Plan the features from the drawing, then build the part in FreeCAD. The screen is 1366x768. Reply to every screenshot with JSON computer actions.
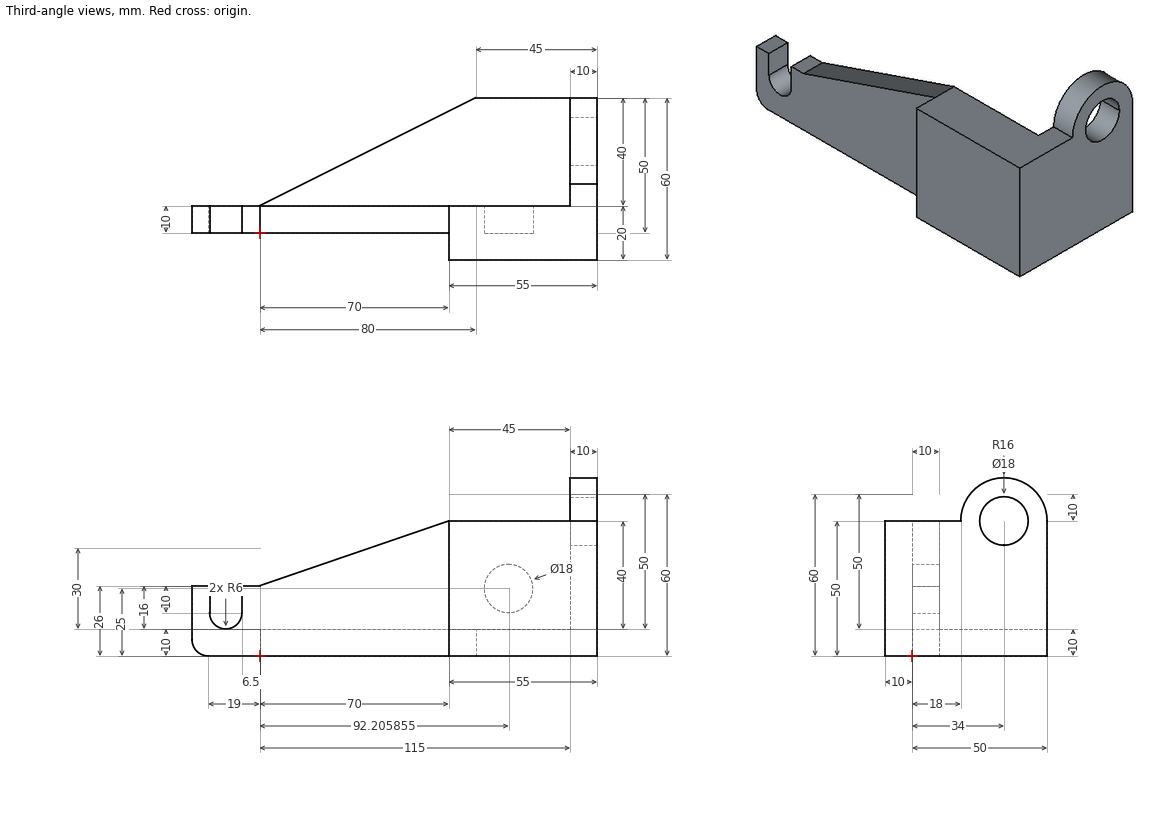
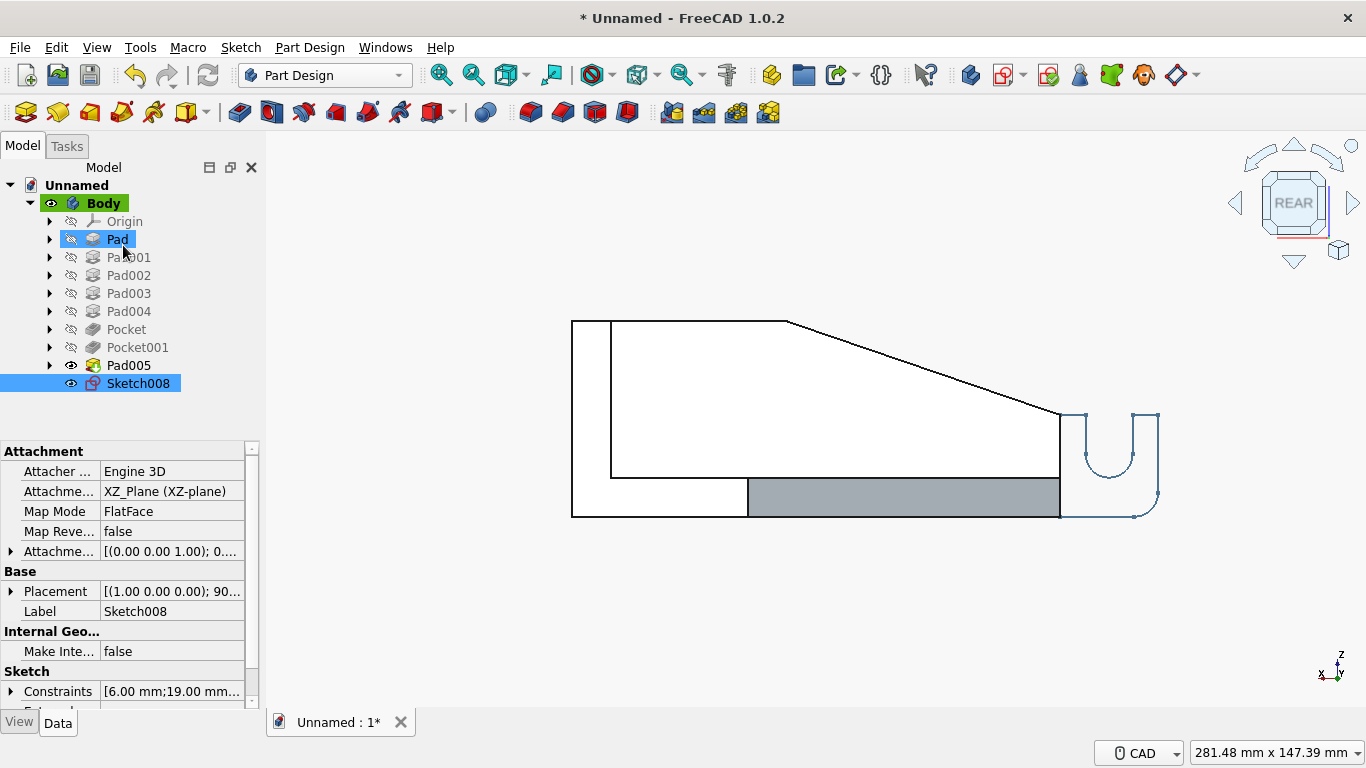
{"action": "left_click", "coordinate": [26, 112]}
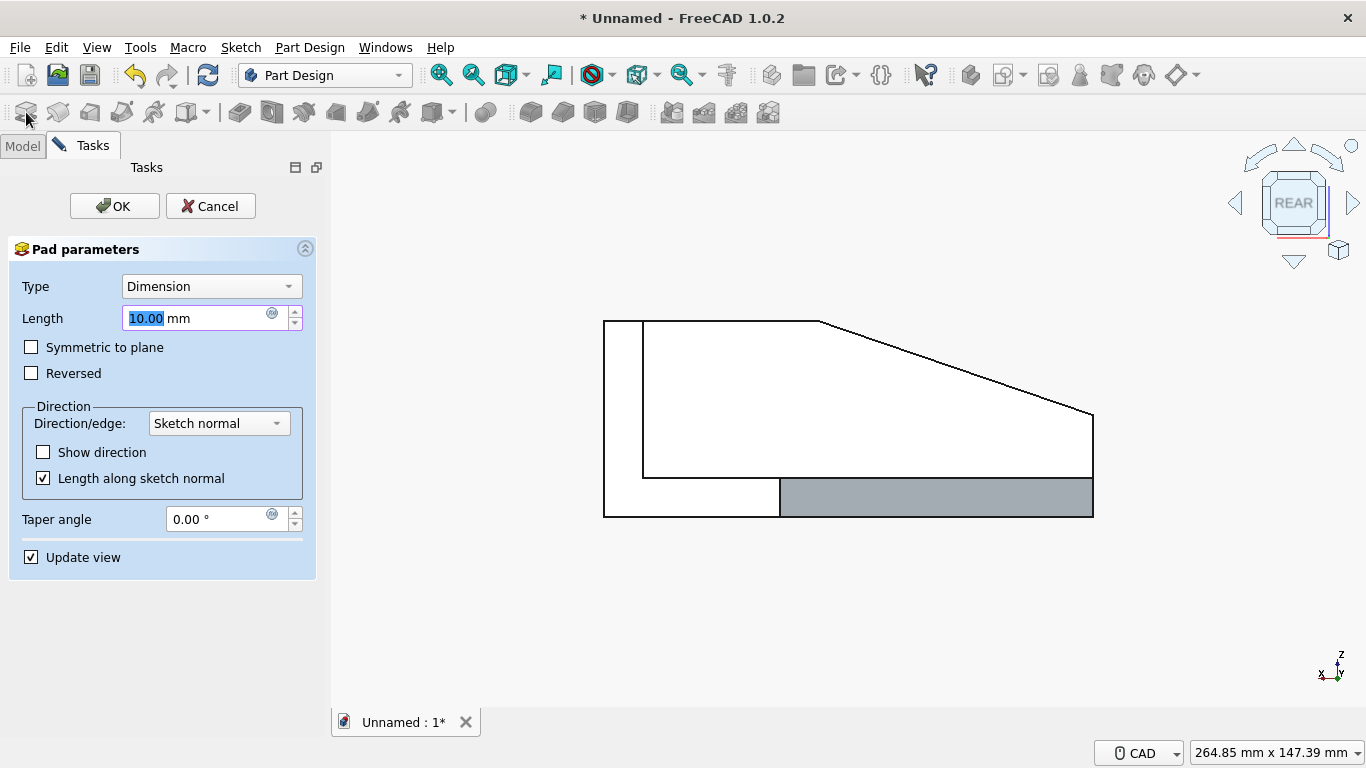
{"action": "type", "text": "10"}
{"action": "key", "text": "Tab"}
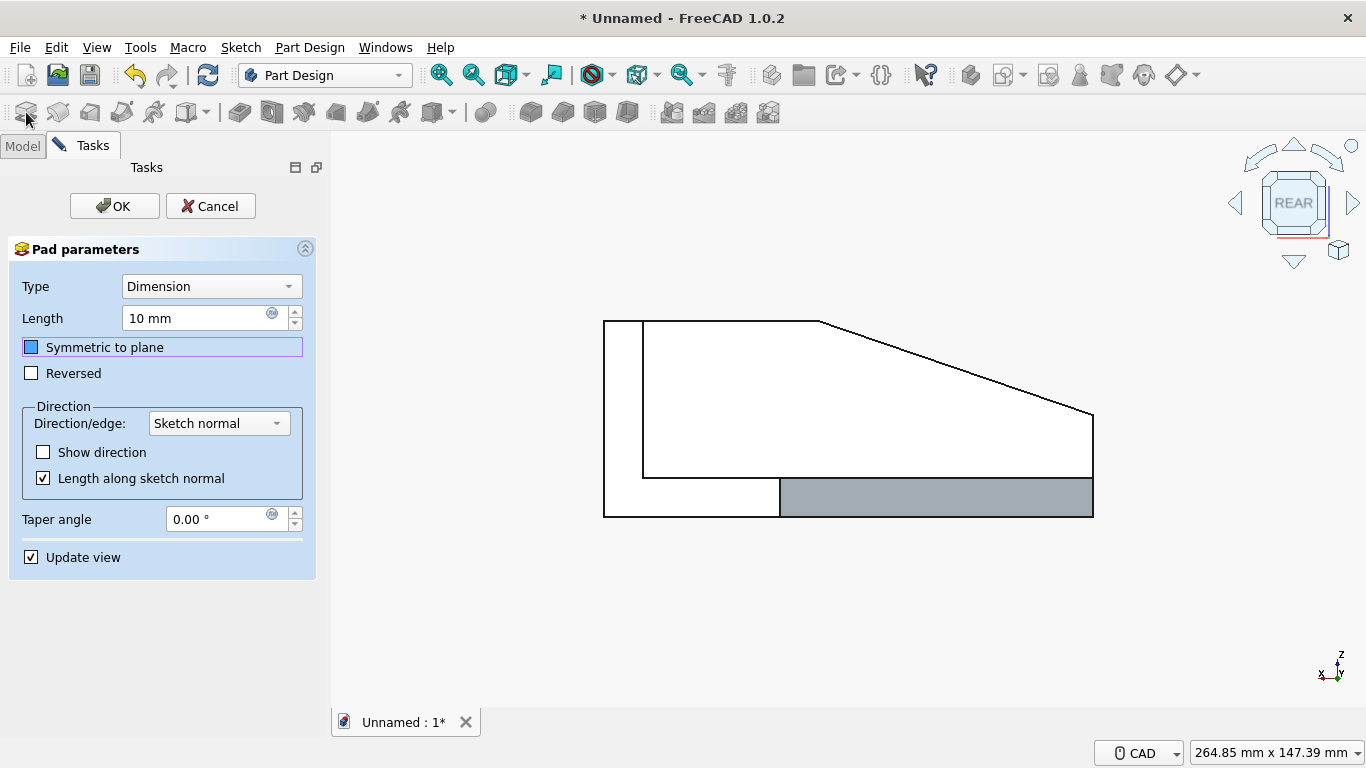
{"action": "left_click", "coordinate": [30, 373]}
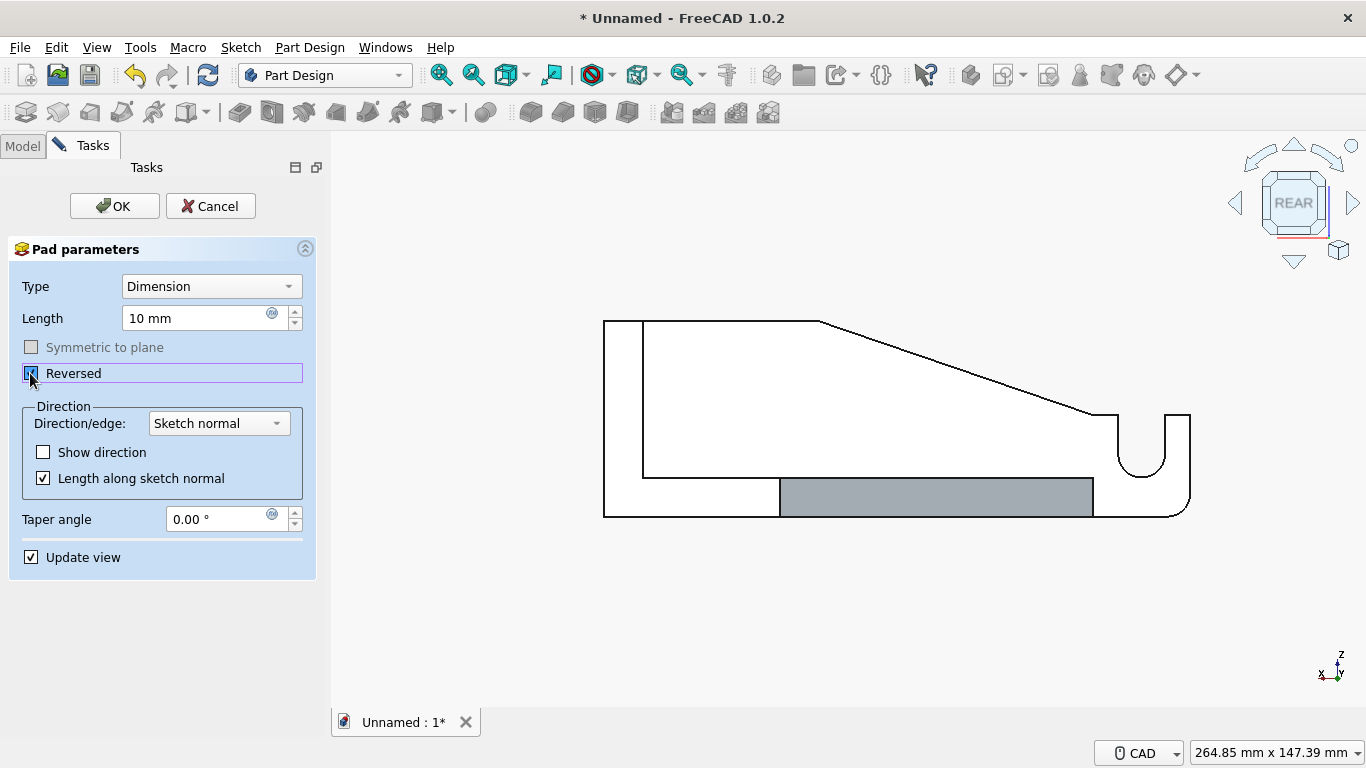
{"action": "left_click", "coordinate": [115, 206]}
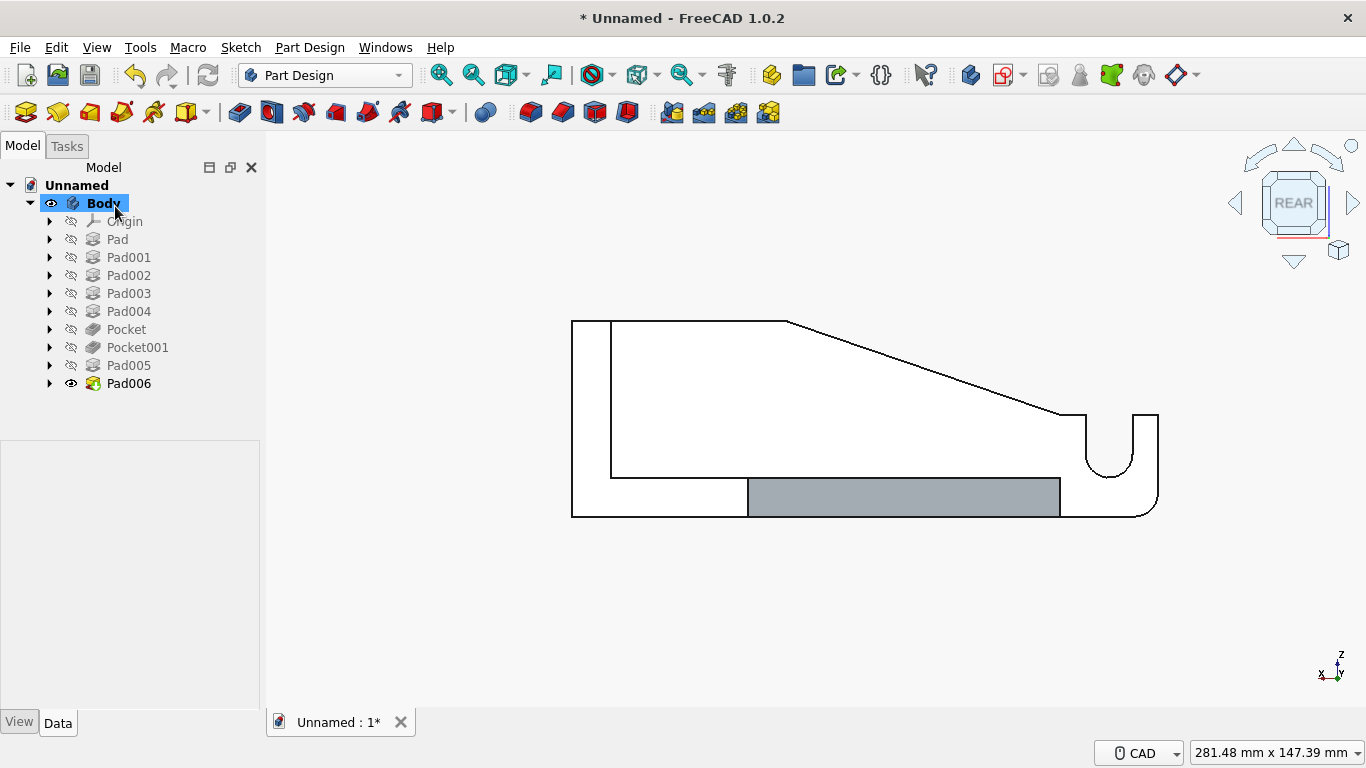
{"action": "key", "text": "0"}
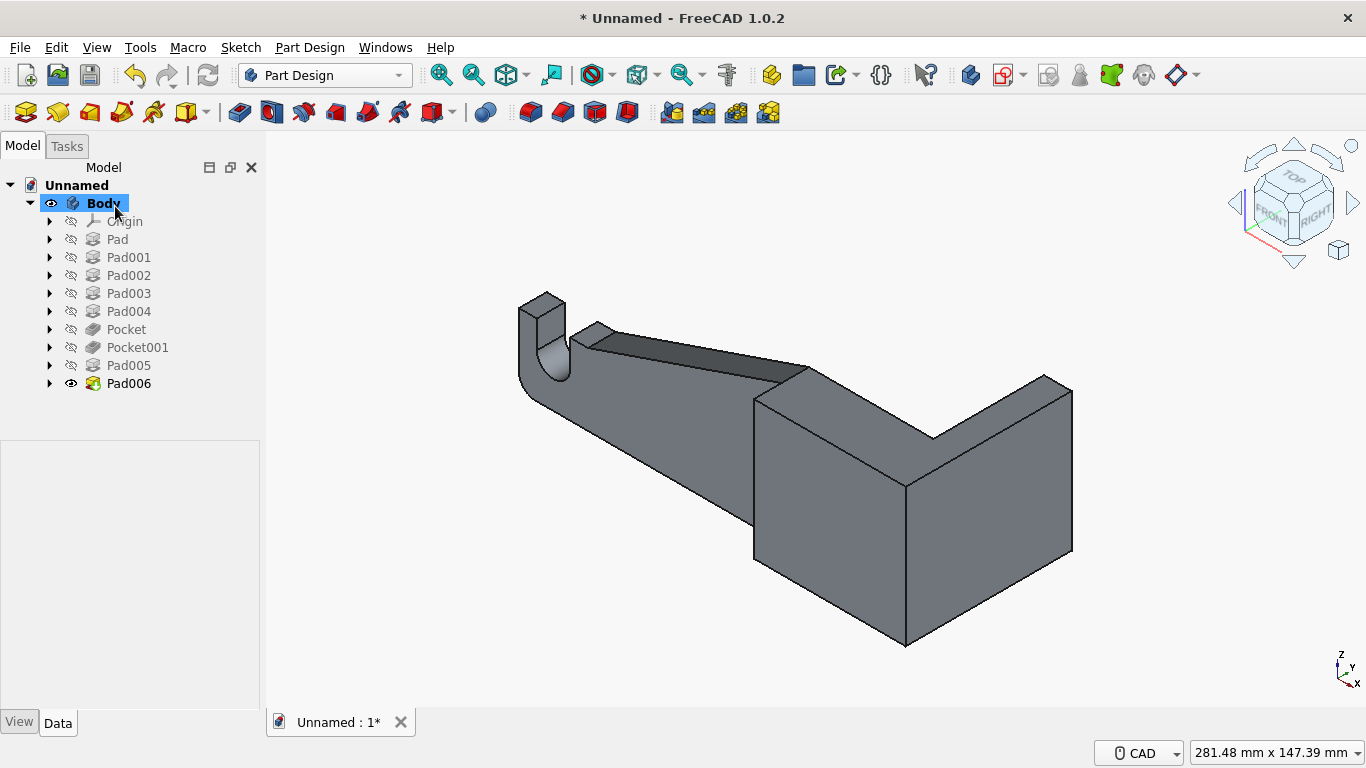
{"action": "left_click", "coordinate": [989, 518]}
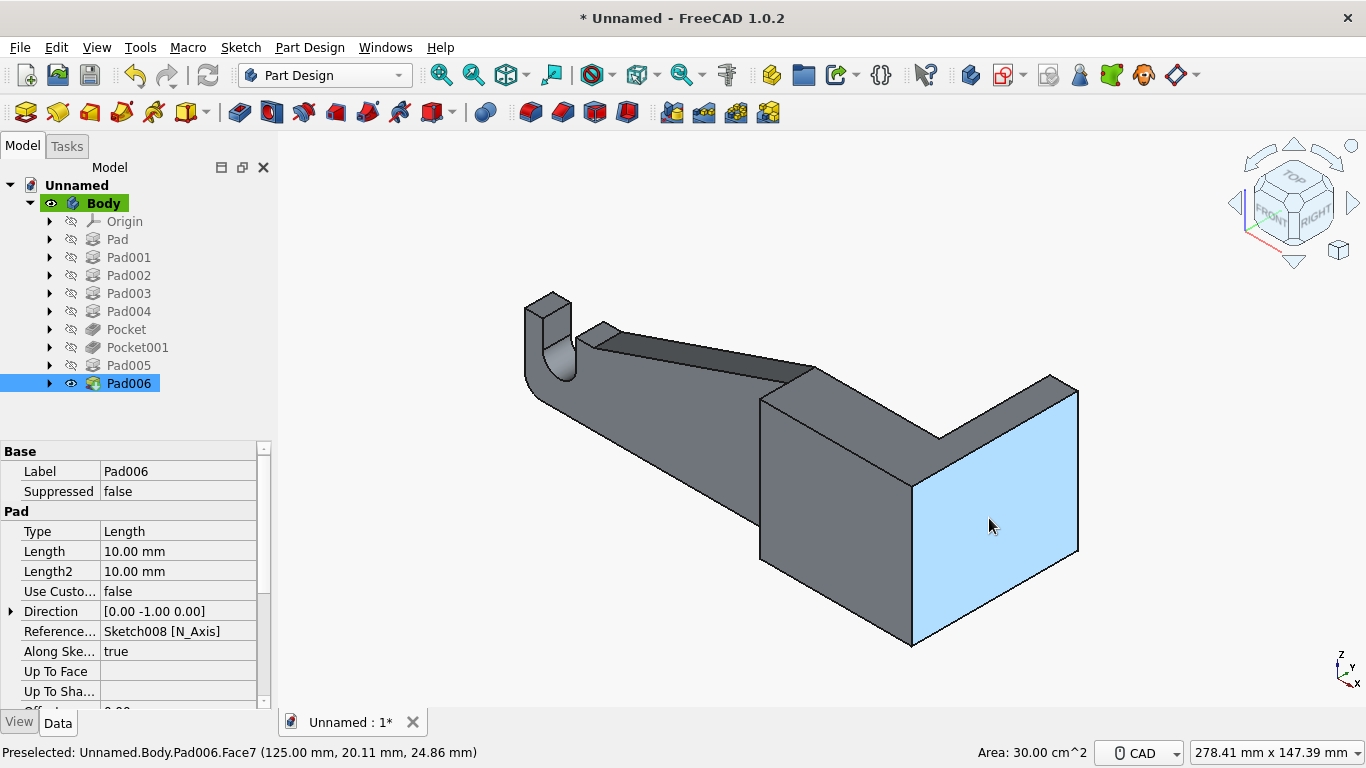
{"action": "left_click", "coordinate": [1004, 76]}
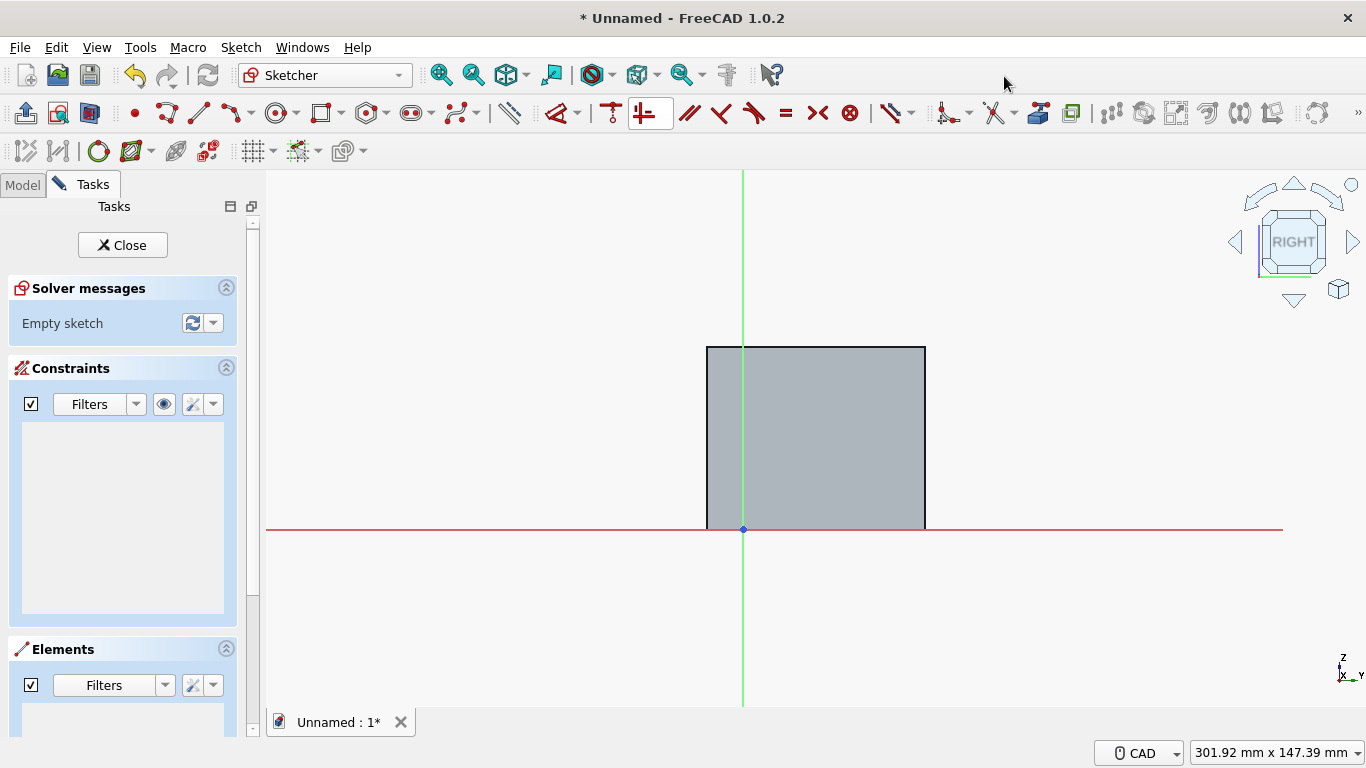
{"action": "scroll", "coordinate": [1011, 350], "scroll_direction": "up", "scroll_amount": 2}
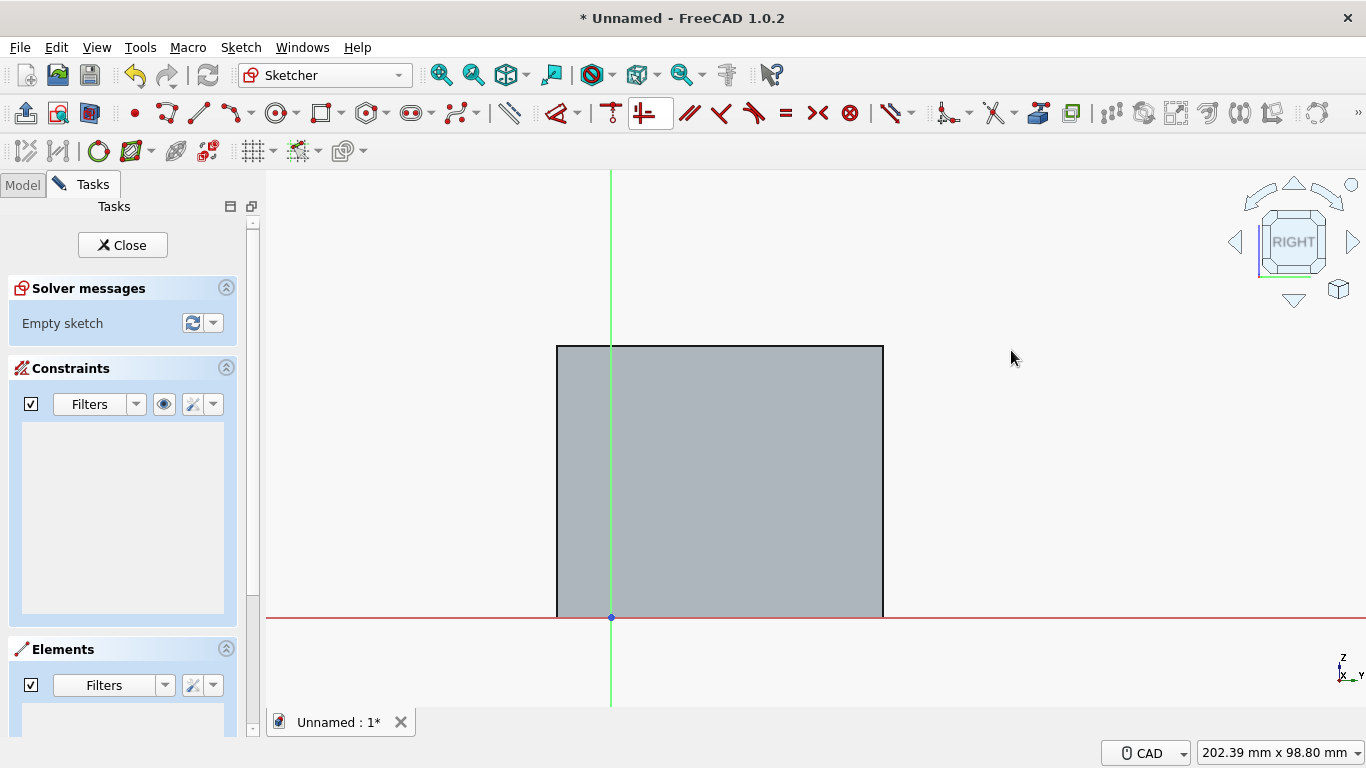
{"action": "left_click", "coordinate": [200, 114]}